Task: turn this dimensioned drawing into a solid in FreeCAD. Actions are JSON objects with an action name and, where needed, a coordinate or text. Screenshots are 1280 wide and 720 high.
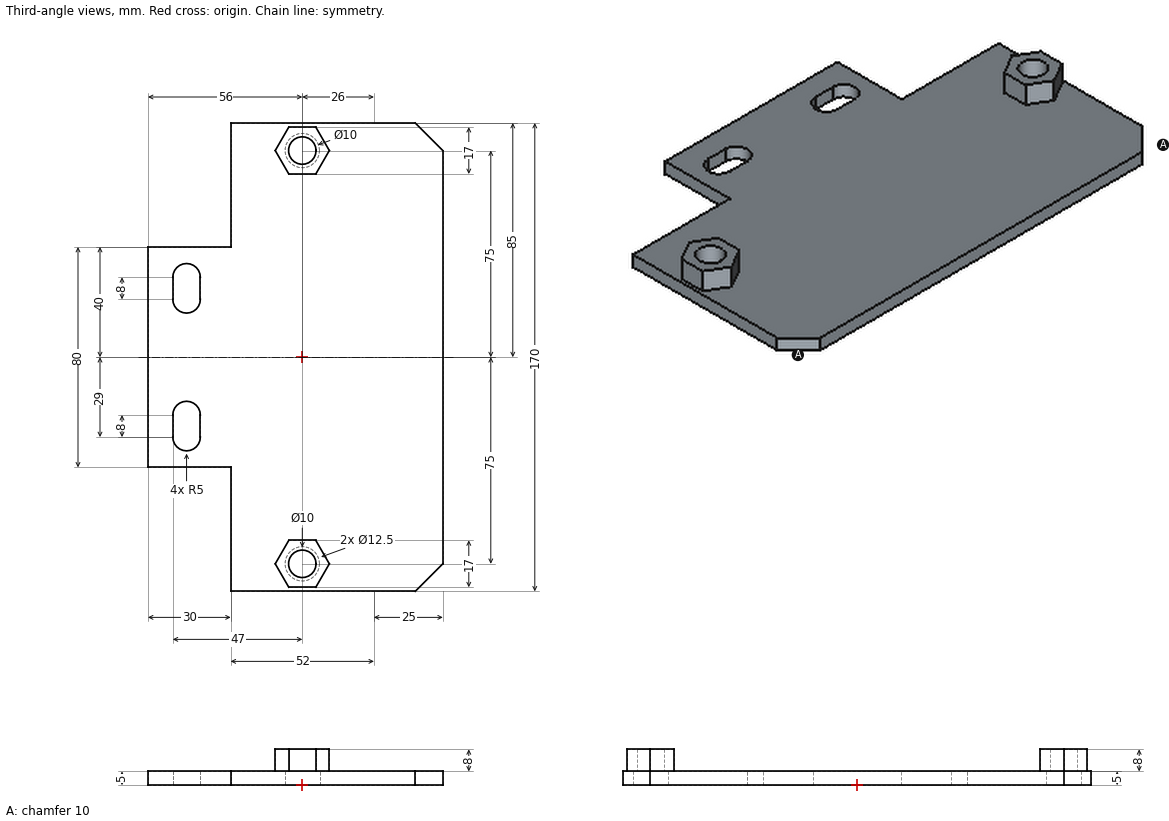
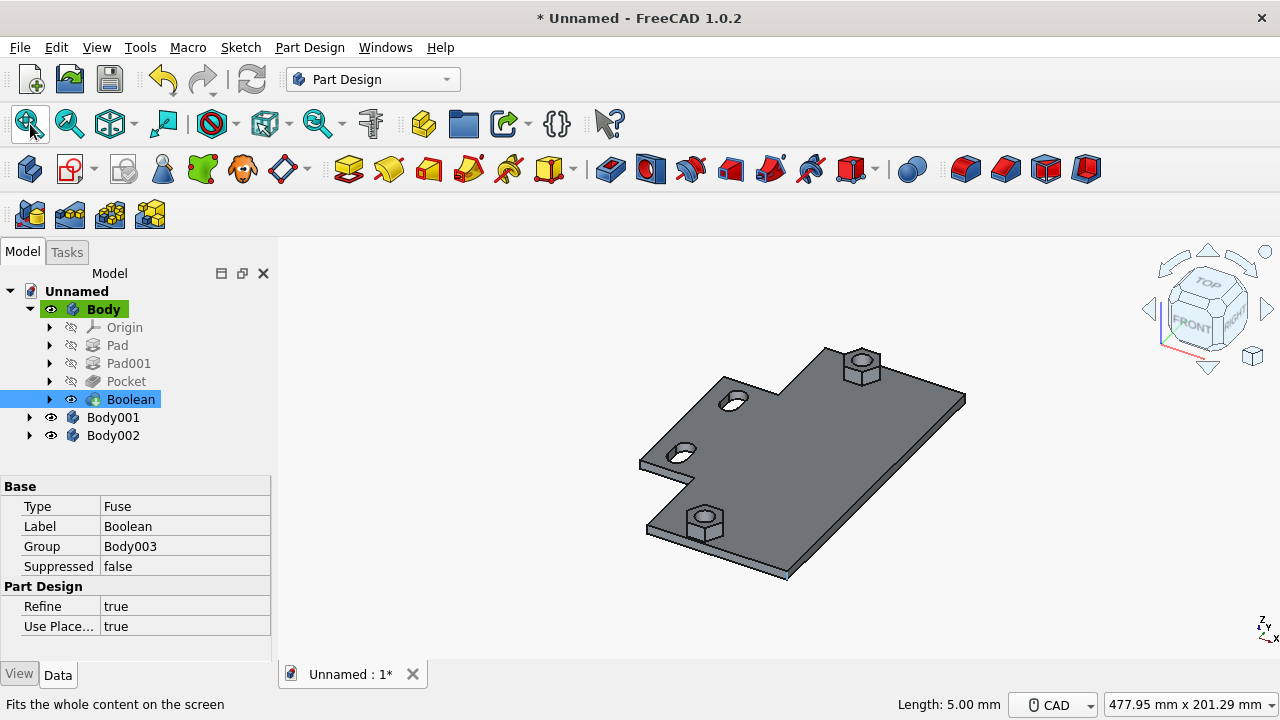
{"action": "key", "text": "0"}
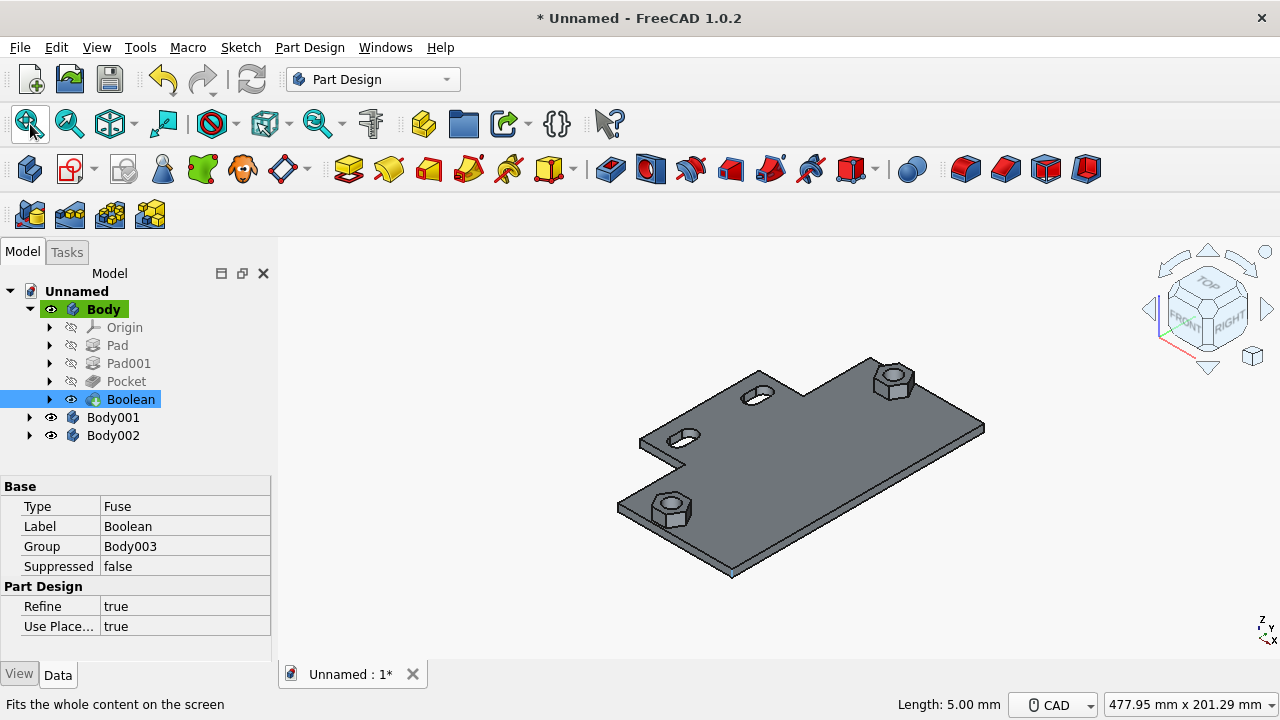
{"action": "scroll", "coordinate": [984, 427], "scroll_direction": "up", "scroll_amount": 7}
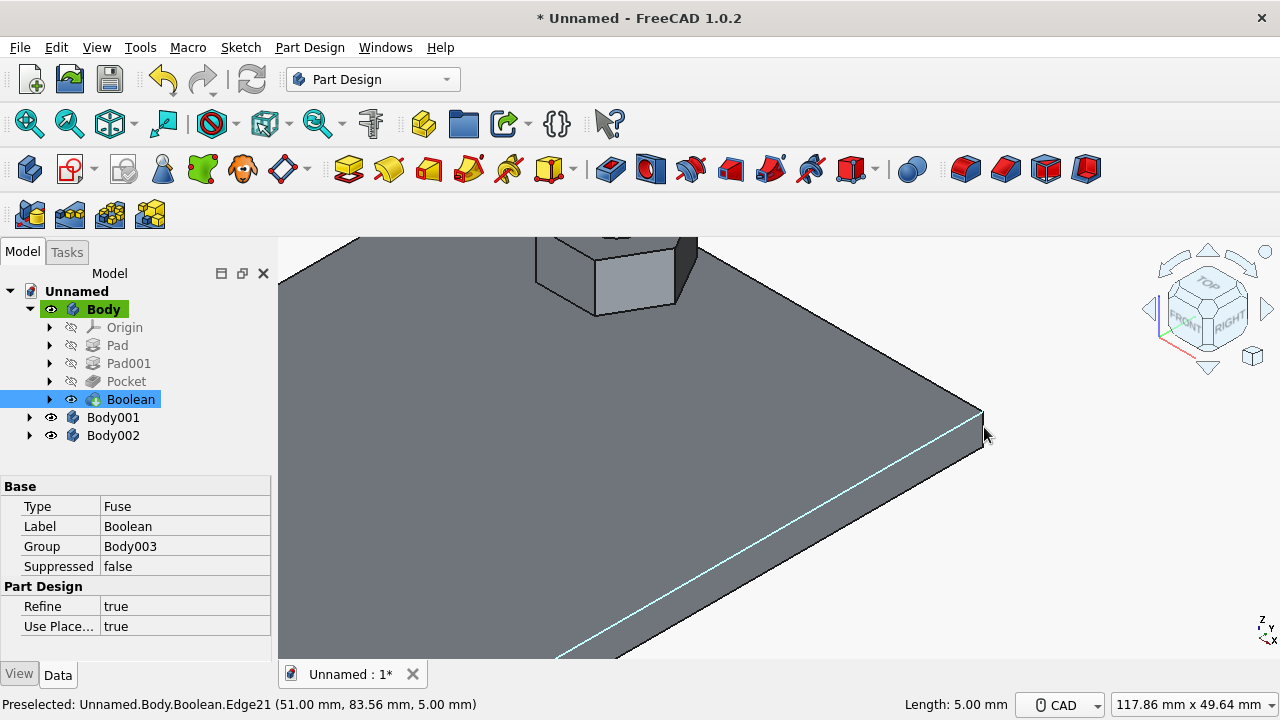
{"action": "left_click", "coordinate": [30, 124]}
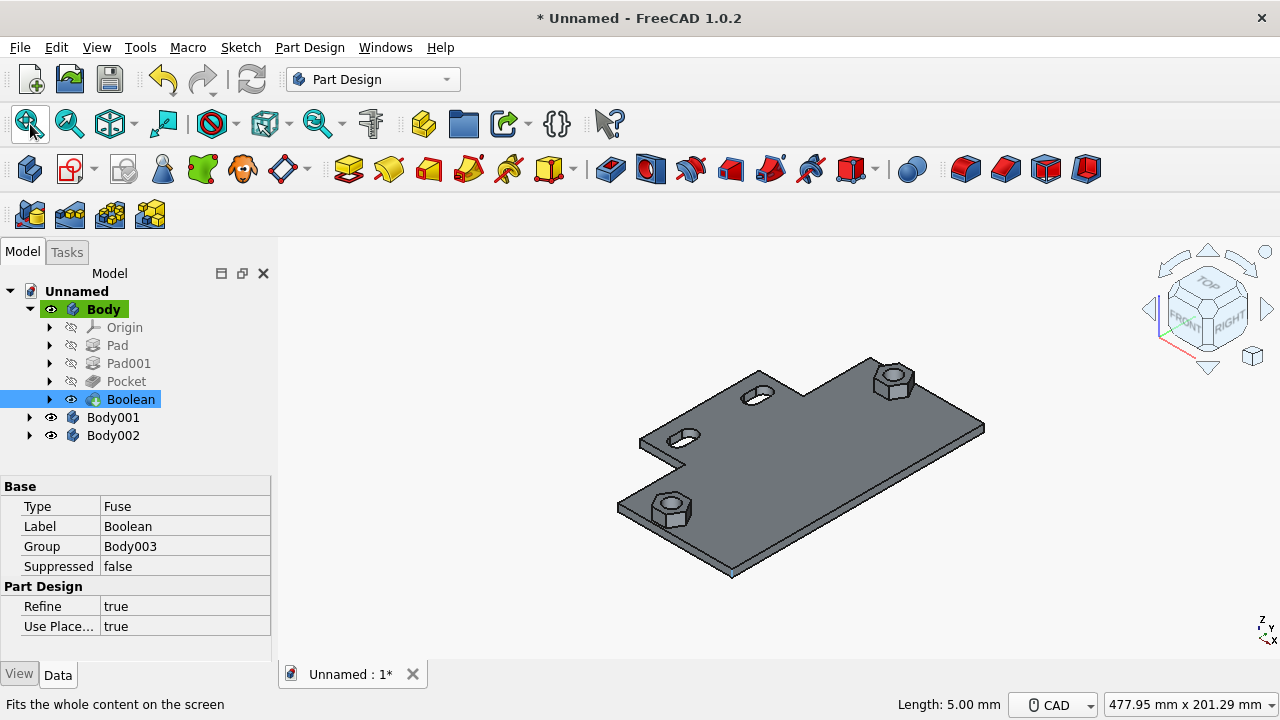
{"action": "key", "text": "2"}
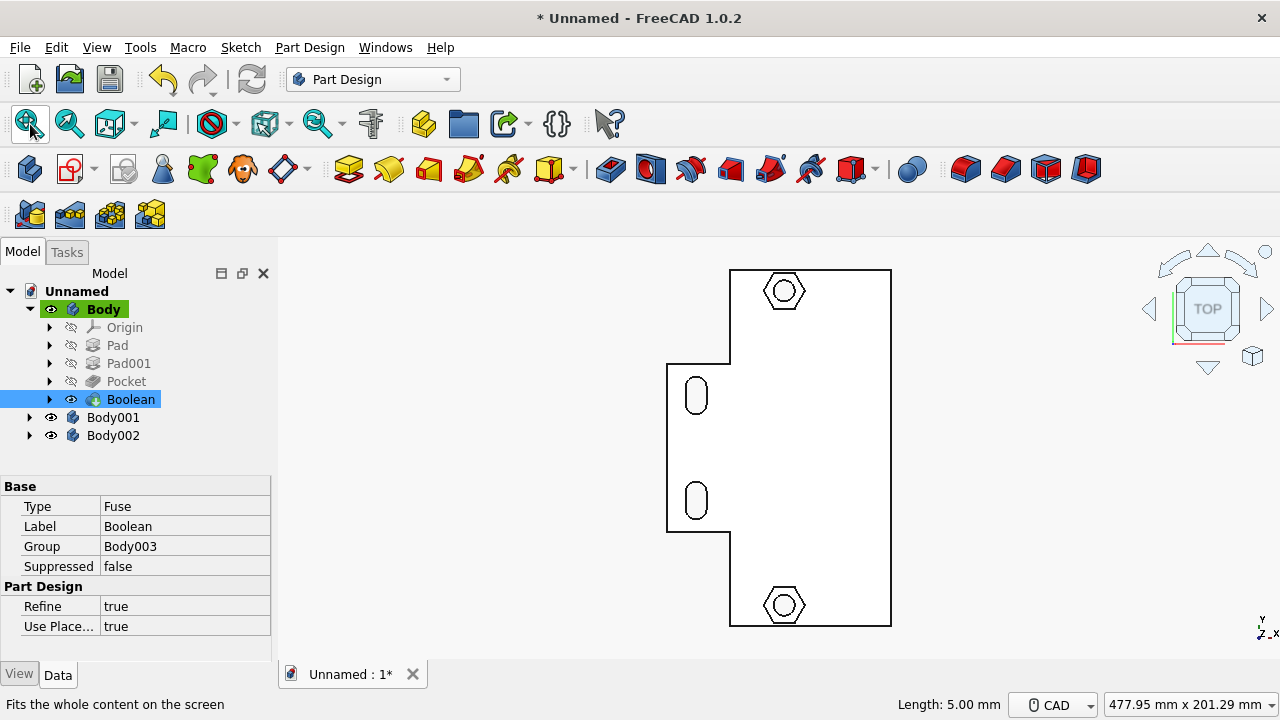
{"action": "scroll", "coordinate": [891, 269], "scroll_direction": "up", "scroll_amount": 7}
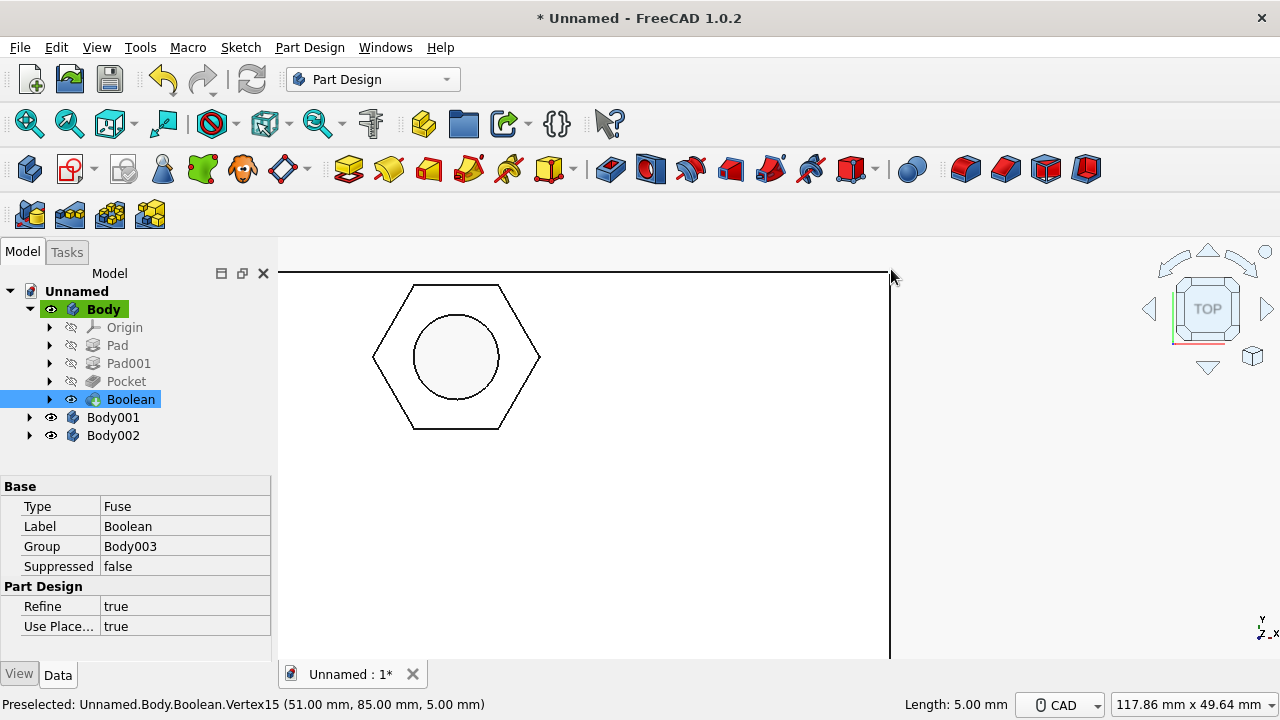
{"action": "left_click", "coordinate": [30, 124]}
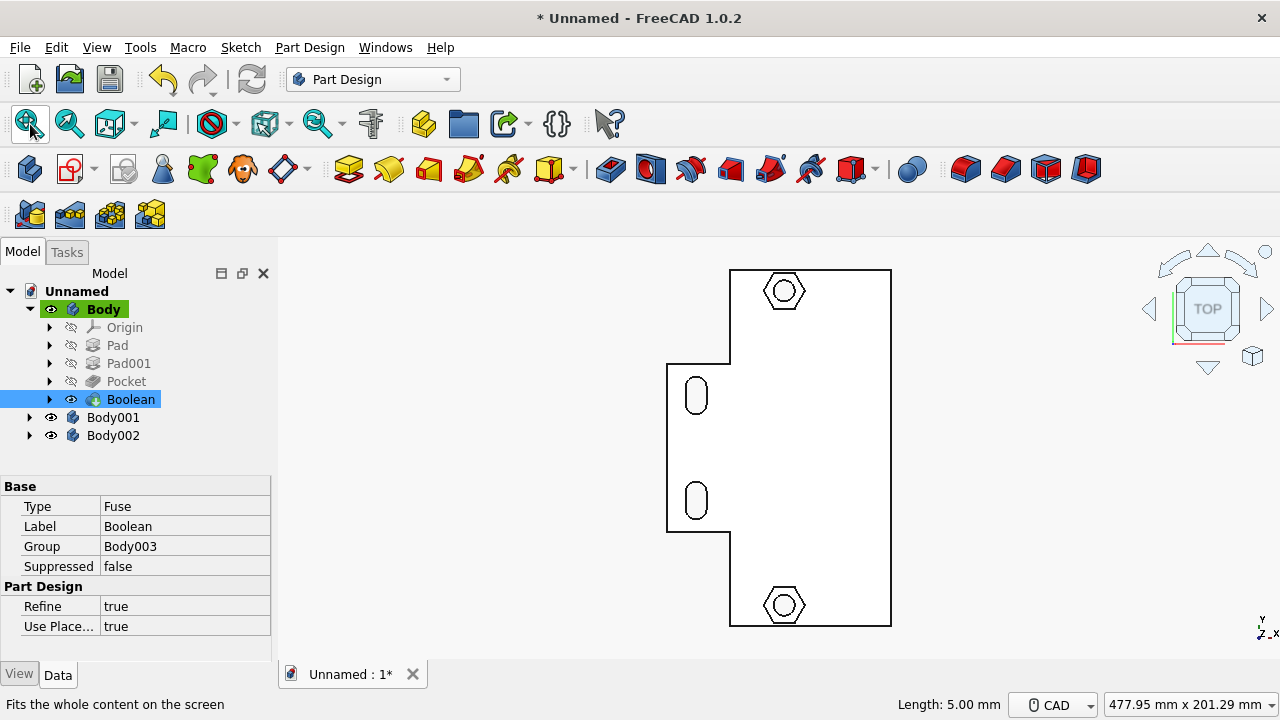
{"action": "key", "text": "1"}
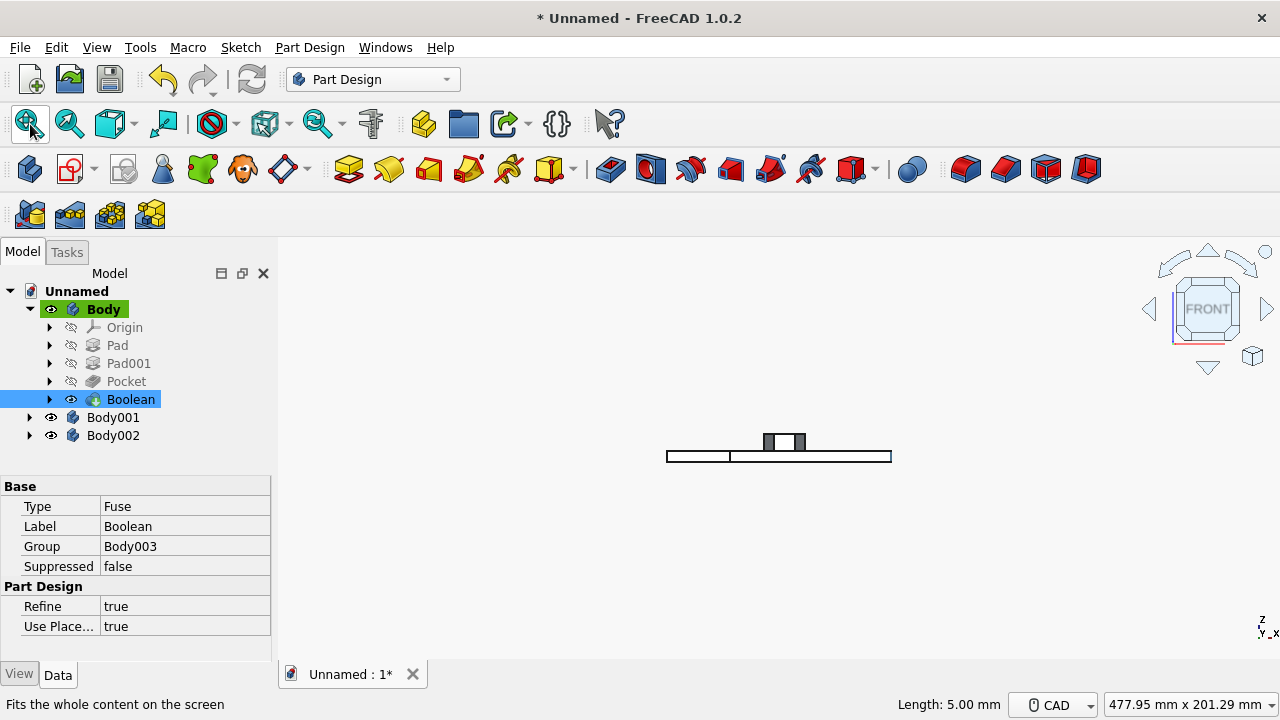
{"action": "left_click", "coordinate": [30, 124]}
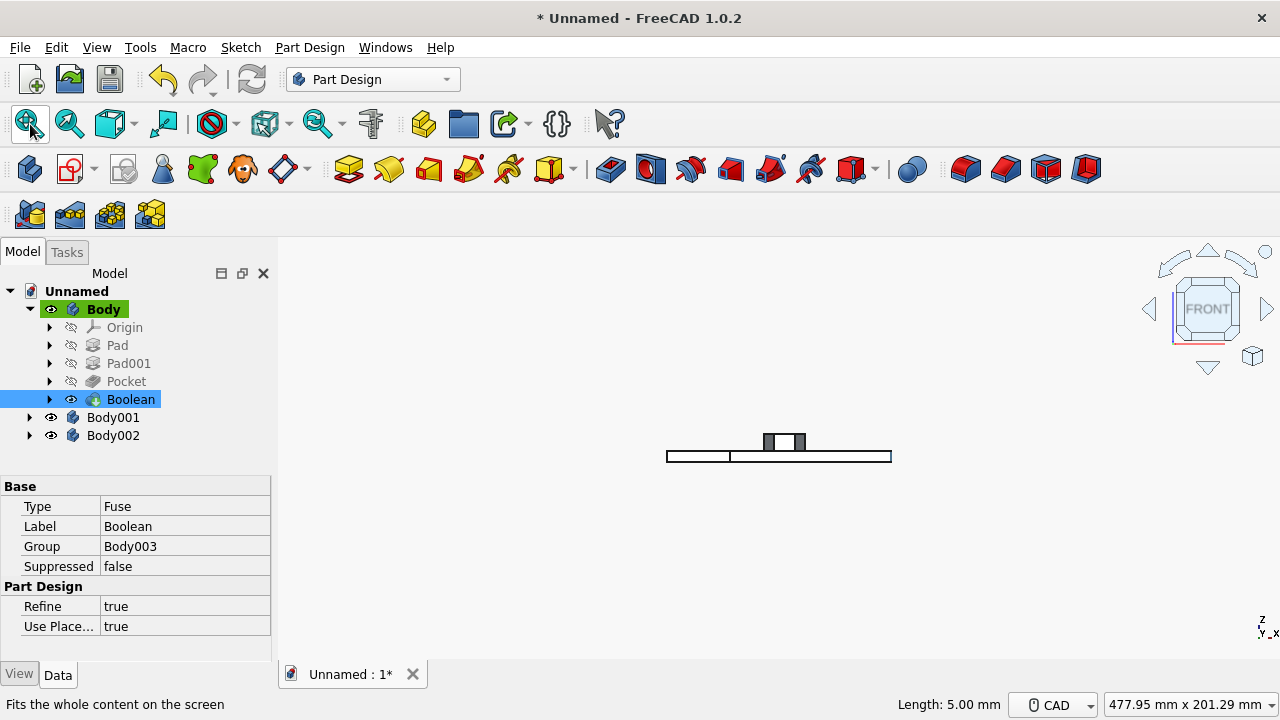
{"action": "scroll", "coordinate": [891, 455], "scroll_direction": "up", "scroll_amount": 7}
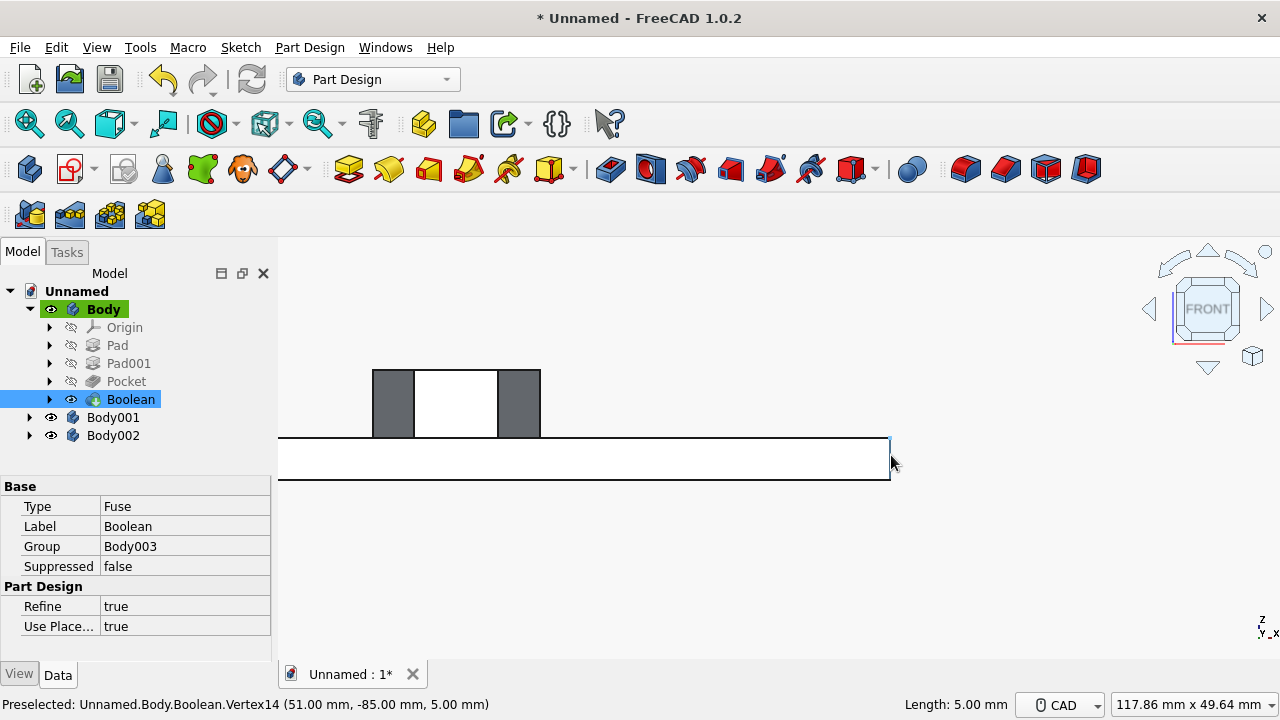
{"action": "left_click", "coordinate": [30, 124]}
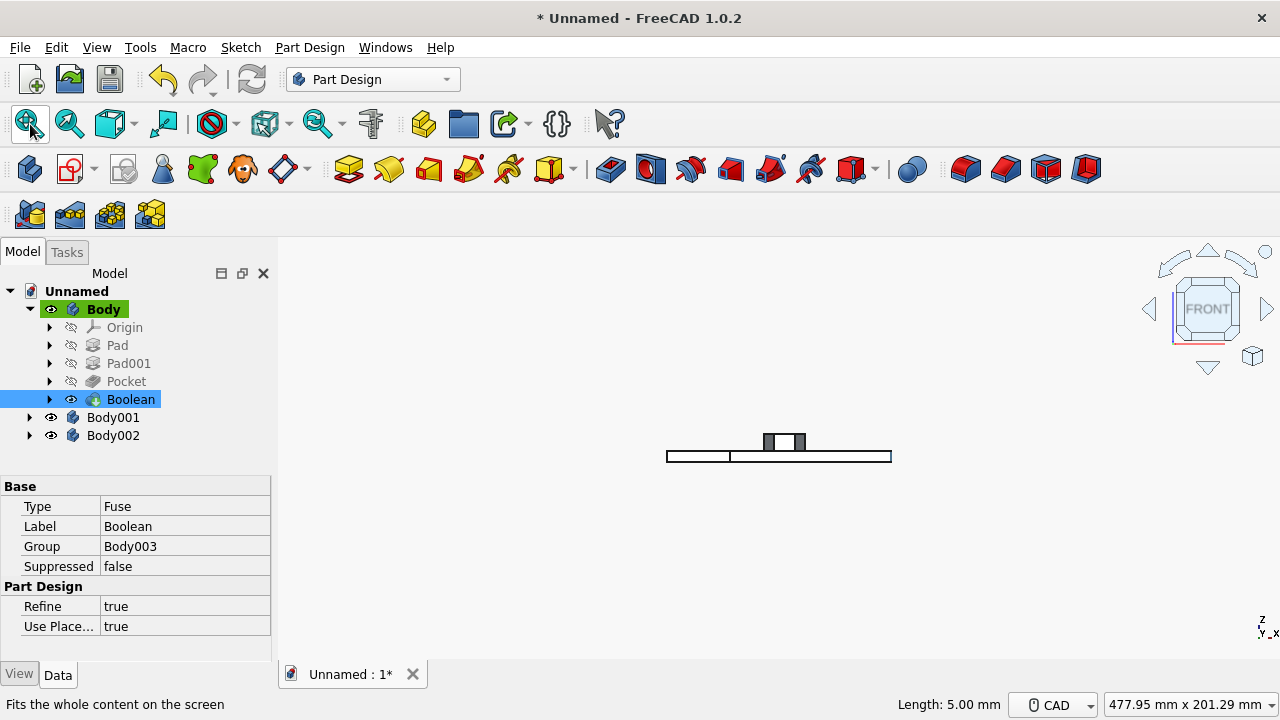
{"action": "key", "text": "3"}